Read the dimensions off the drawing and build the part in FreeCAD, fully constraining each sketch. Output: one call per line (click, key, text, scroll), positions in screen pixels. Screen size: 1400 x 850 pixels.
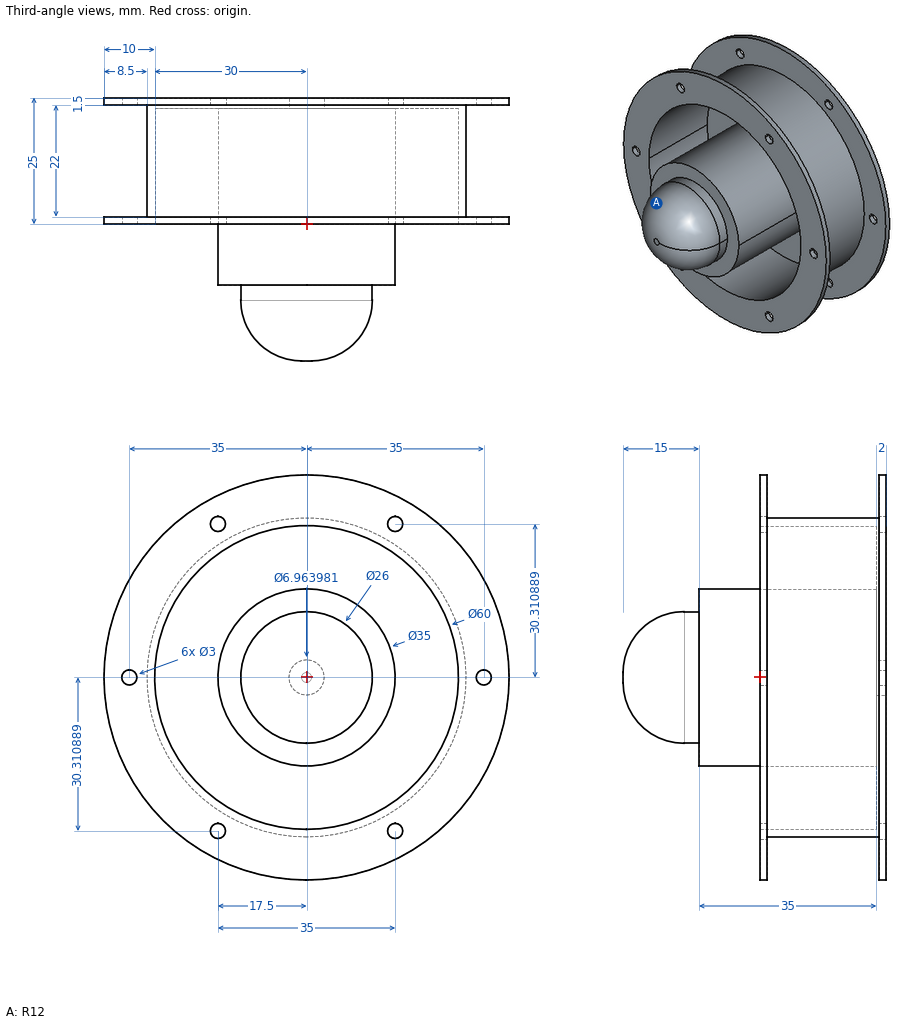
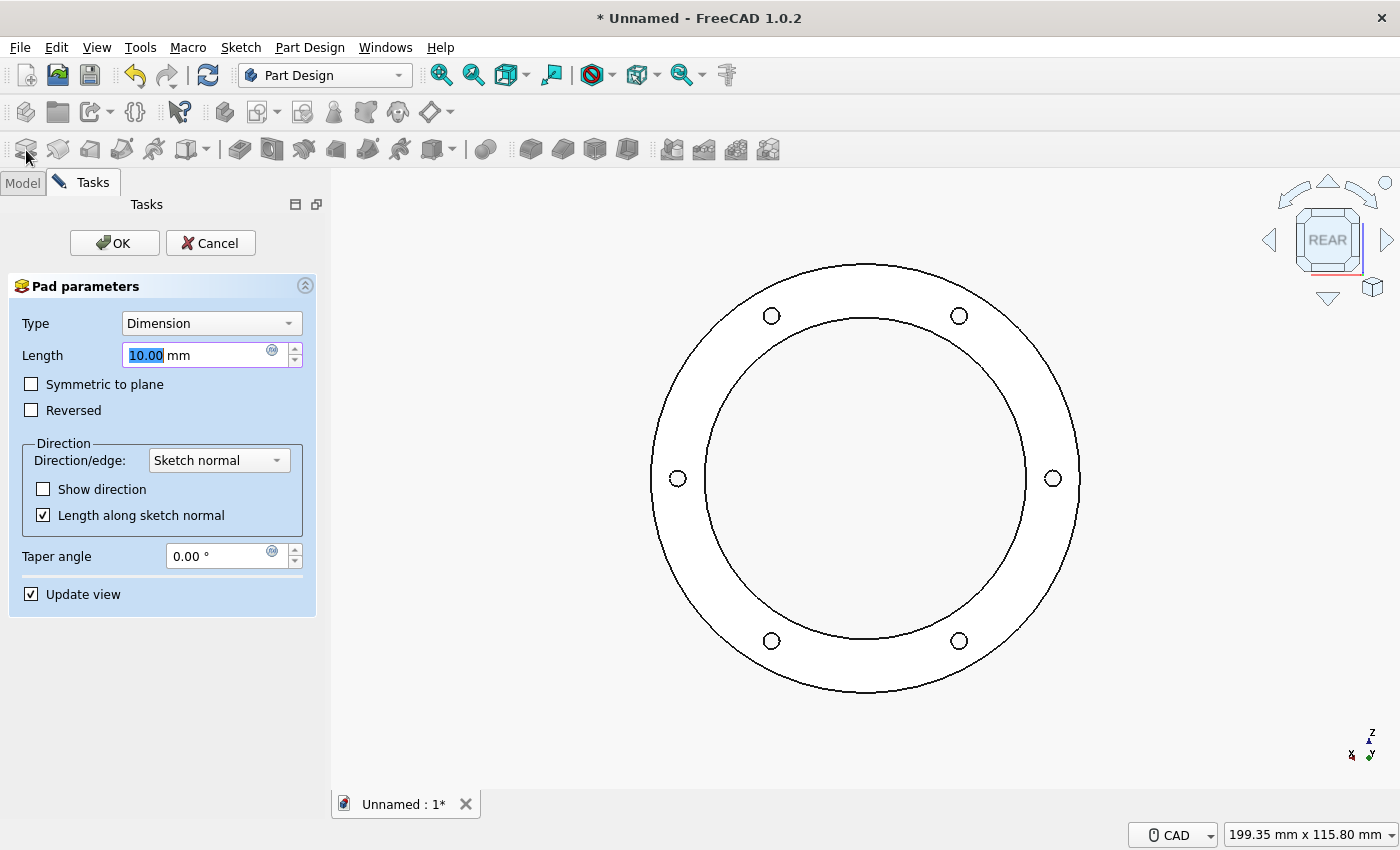
text(2)
key(Tab)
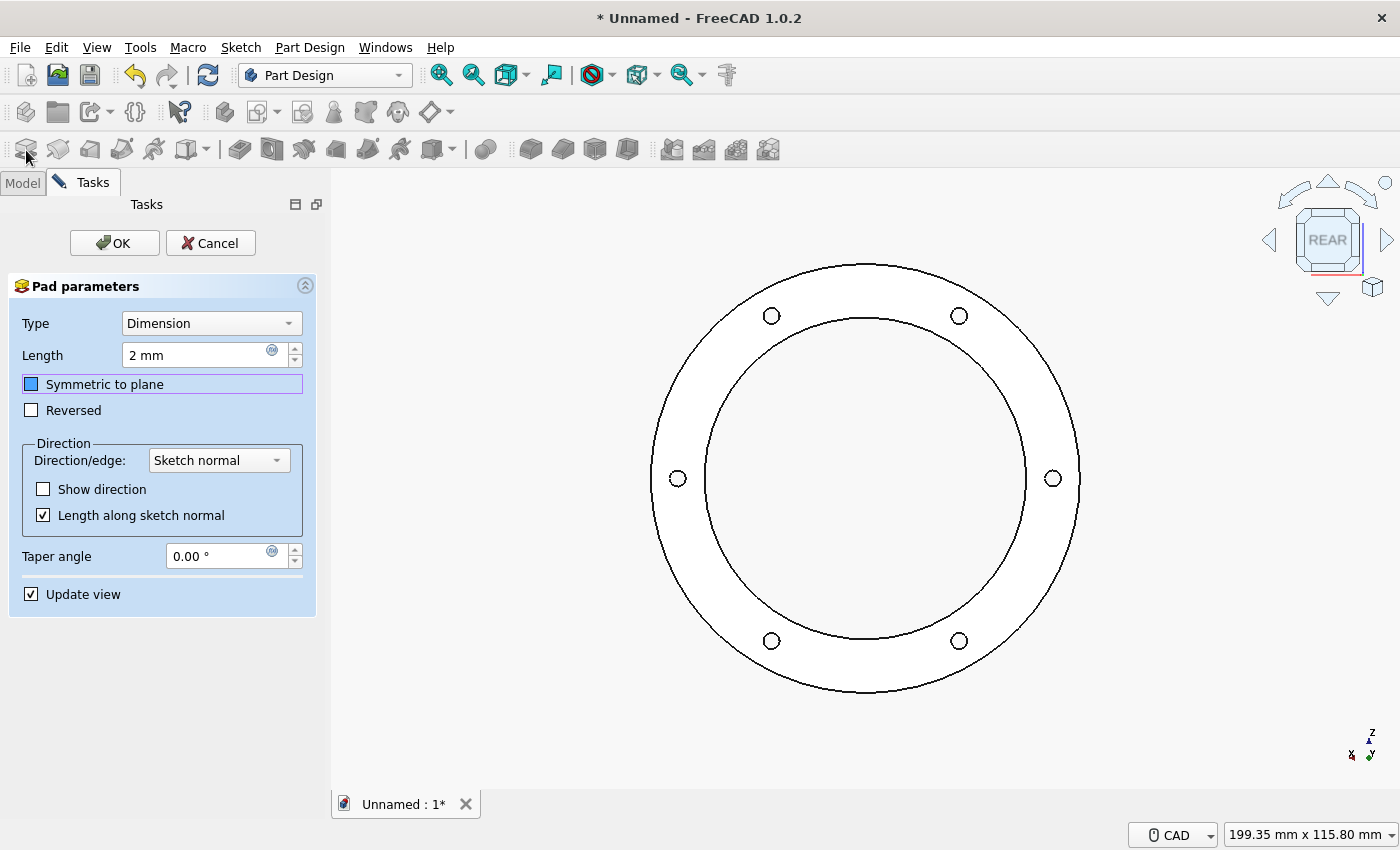
click(30, 410)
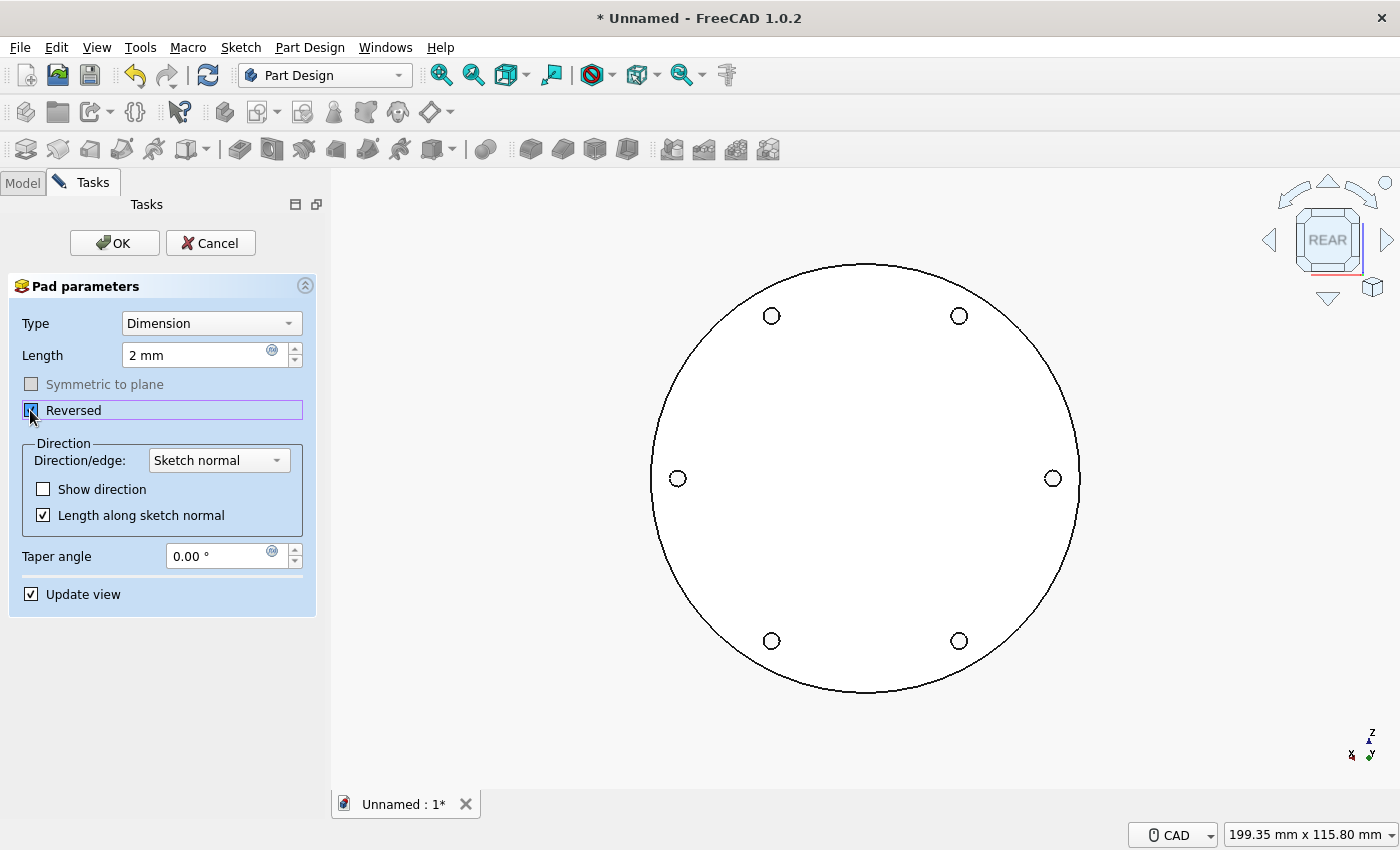
click(115, 243)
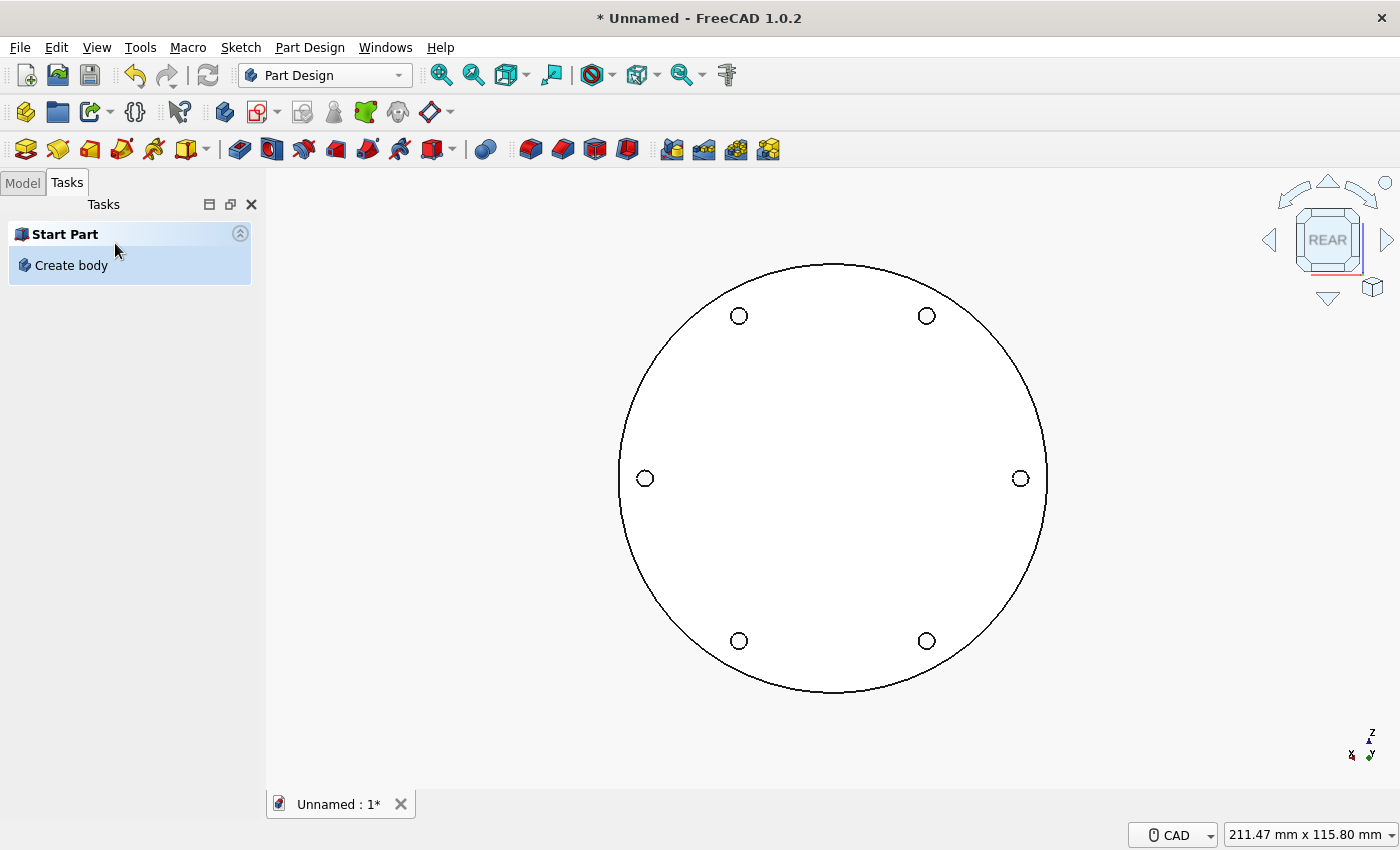
key(0)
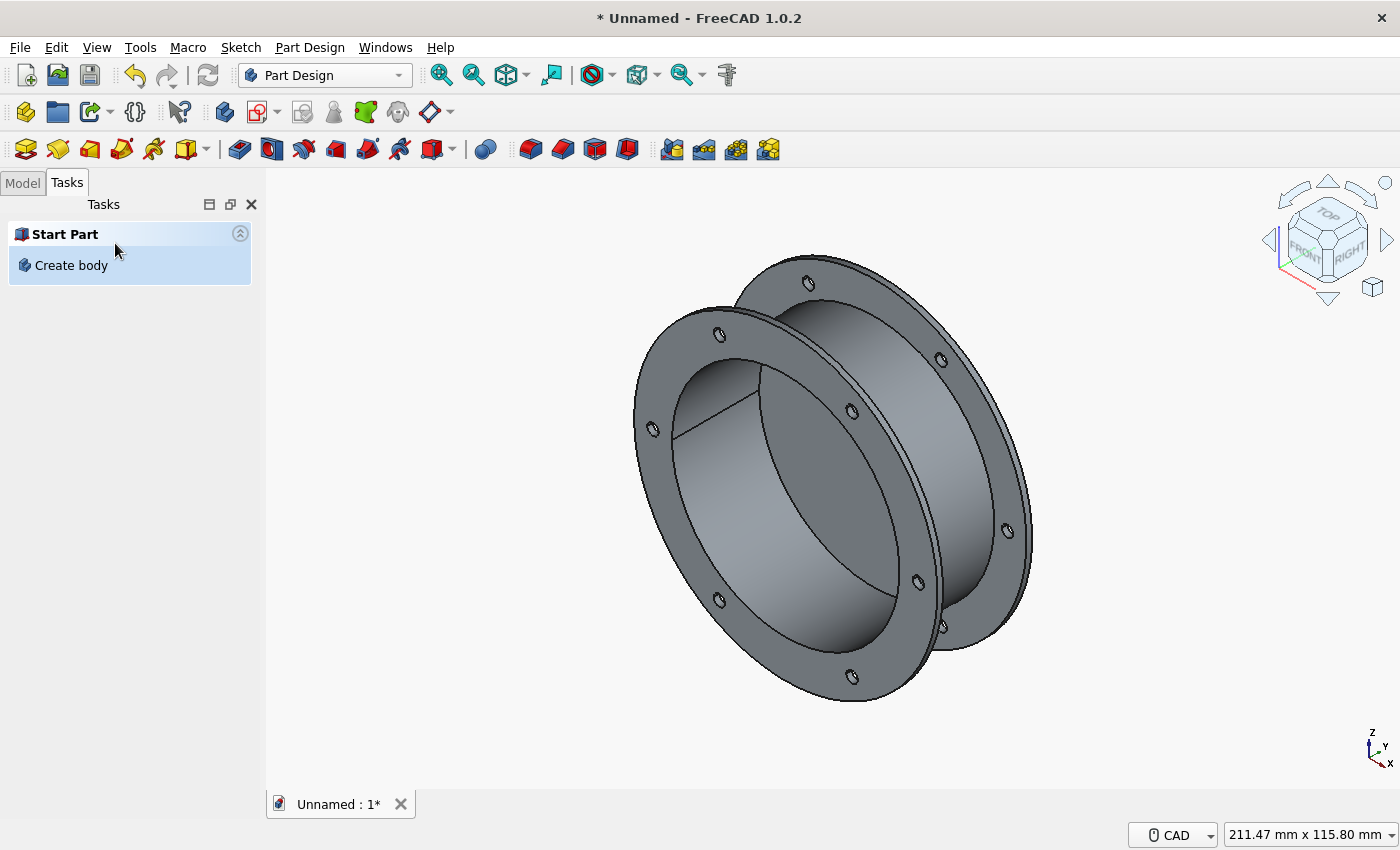
click(840, 436)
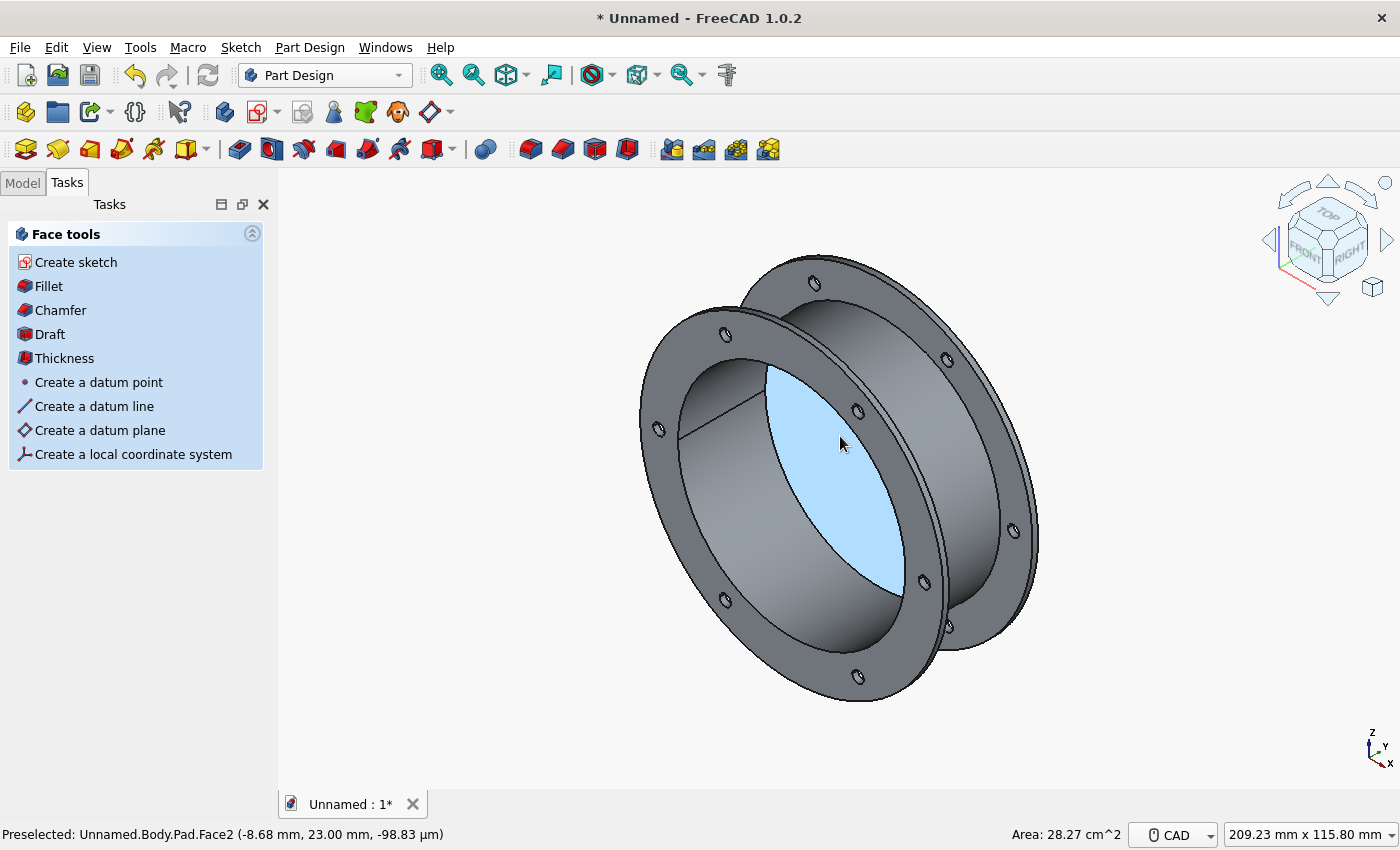
click(258, 112)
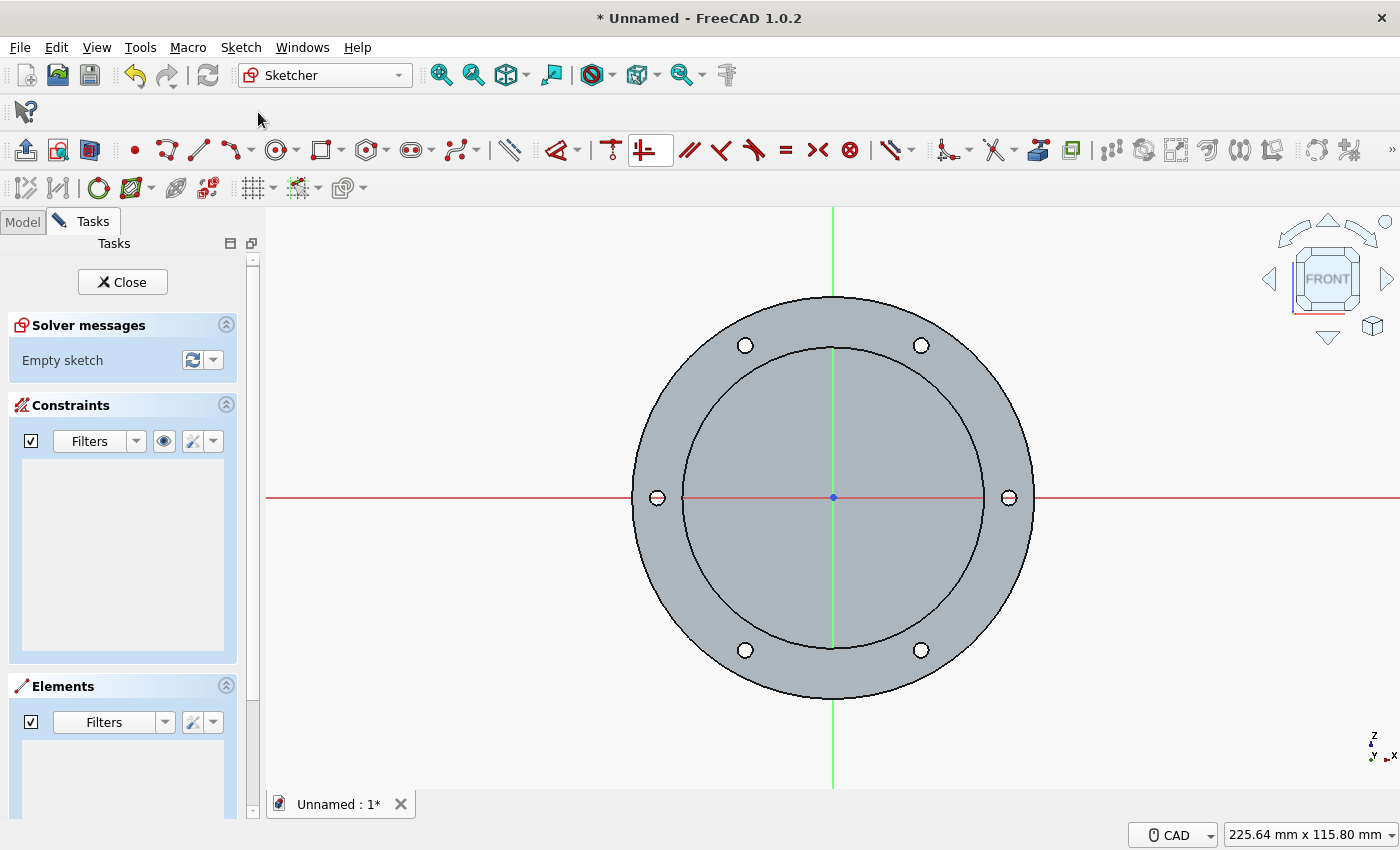
click(90, 150)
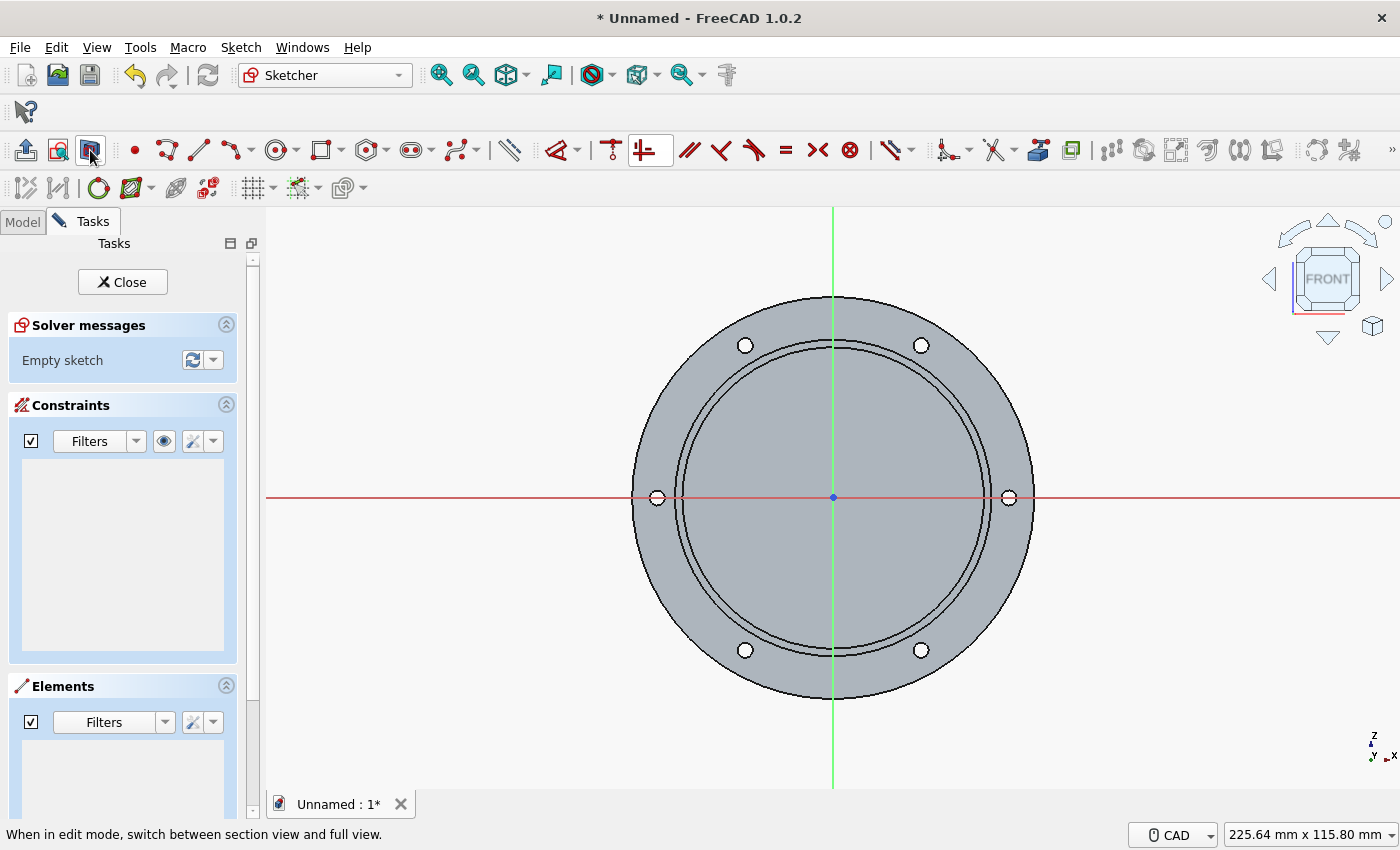
scroll(840, 498, up, 12)